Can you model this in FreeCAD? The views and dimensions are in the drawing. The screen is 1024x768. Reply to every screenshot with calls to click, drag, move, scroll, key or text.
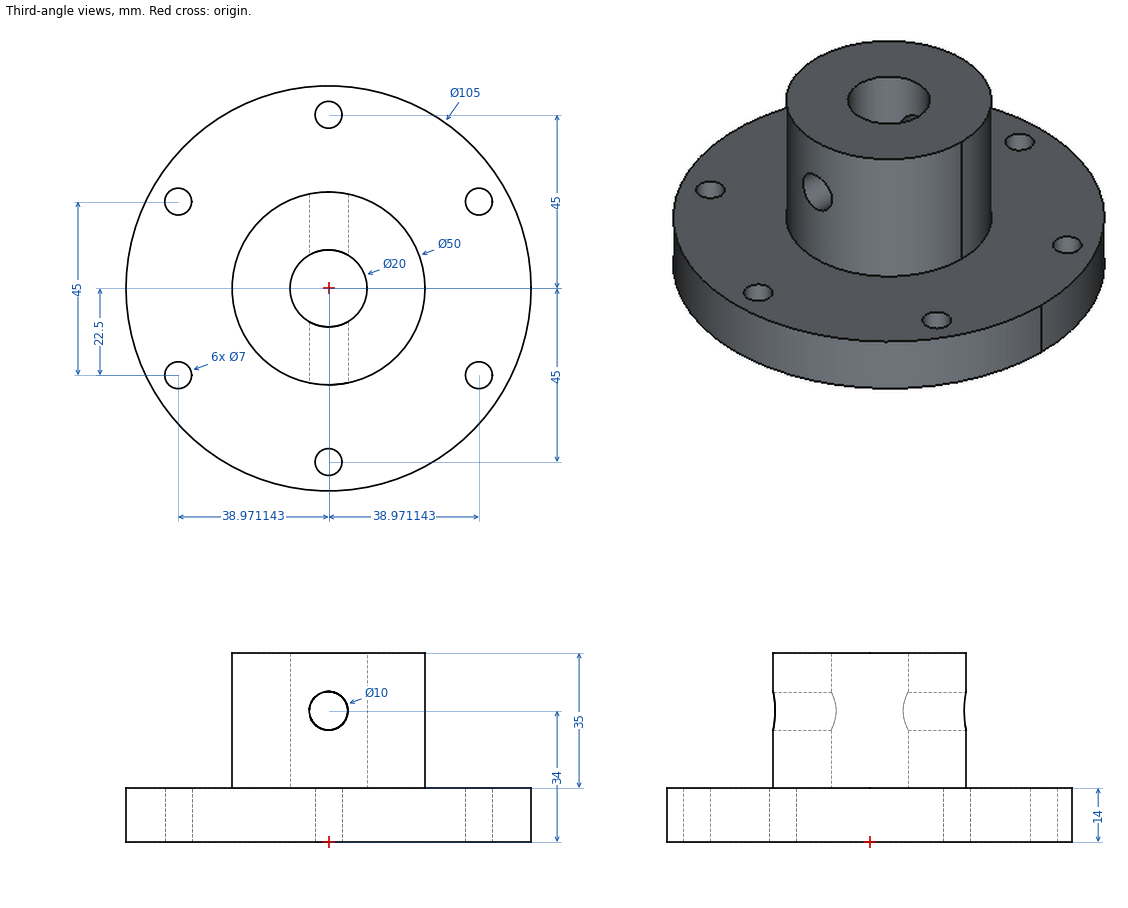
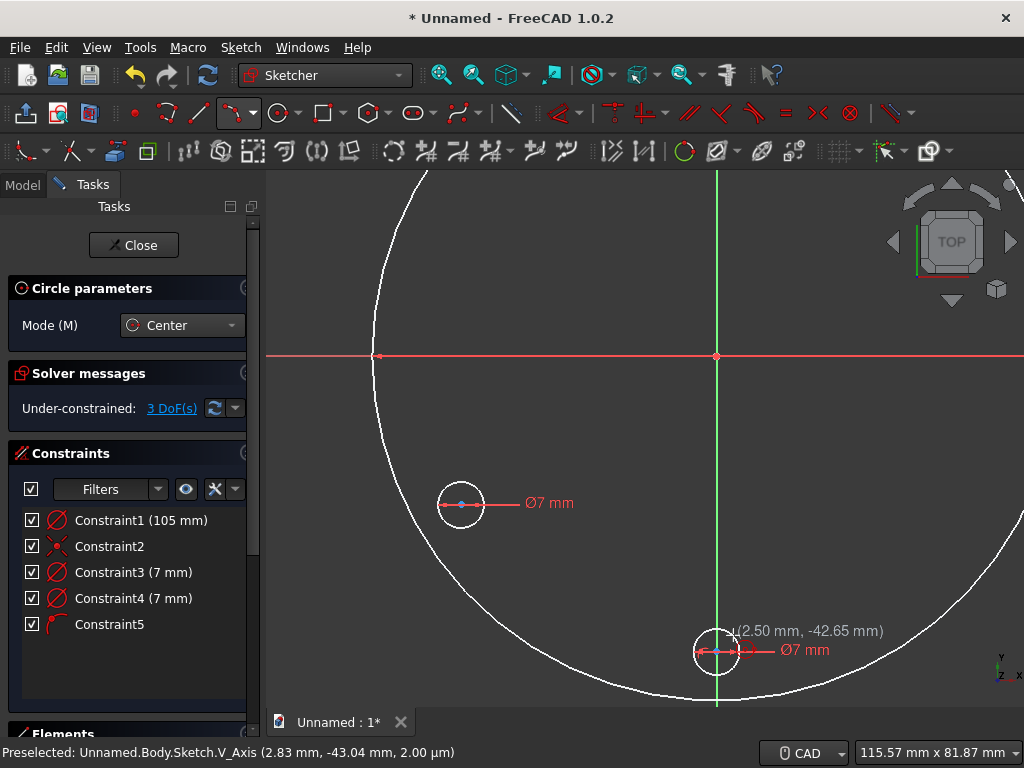
scroll(462, 506, down, 4)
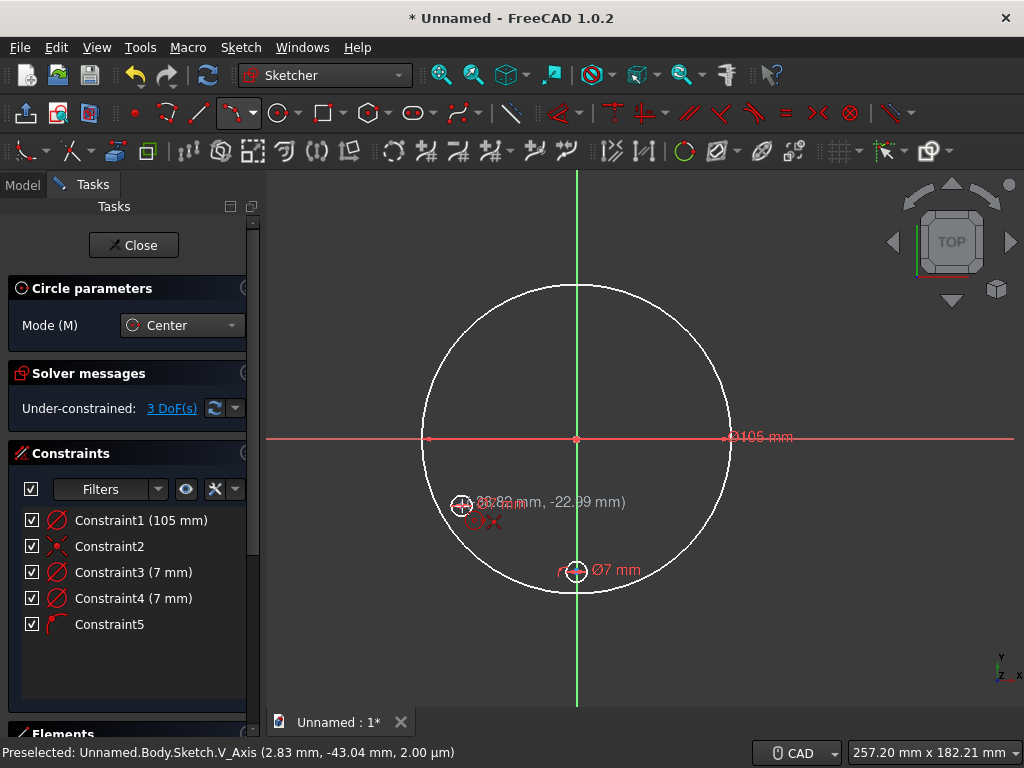
scroll(691, 505, up, 4)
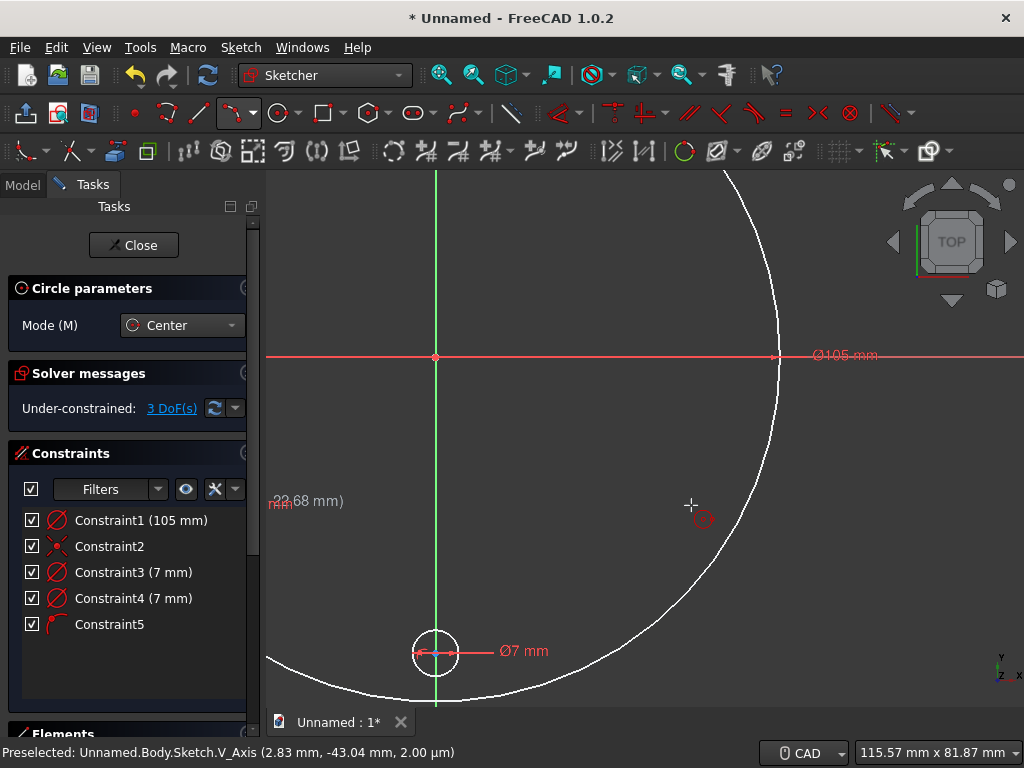
click(691, 505)
move(707, 489)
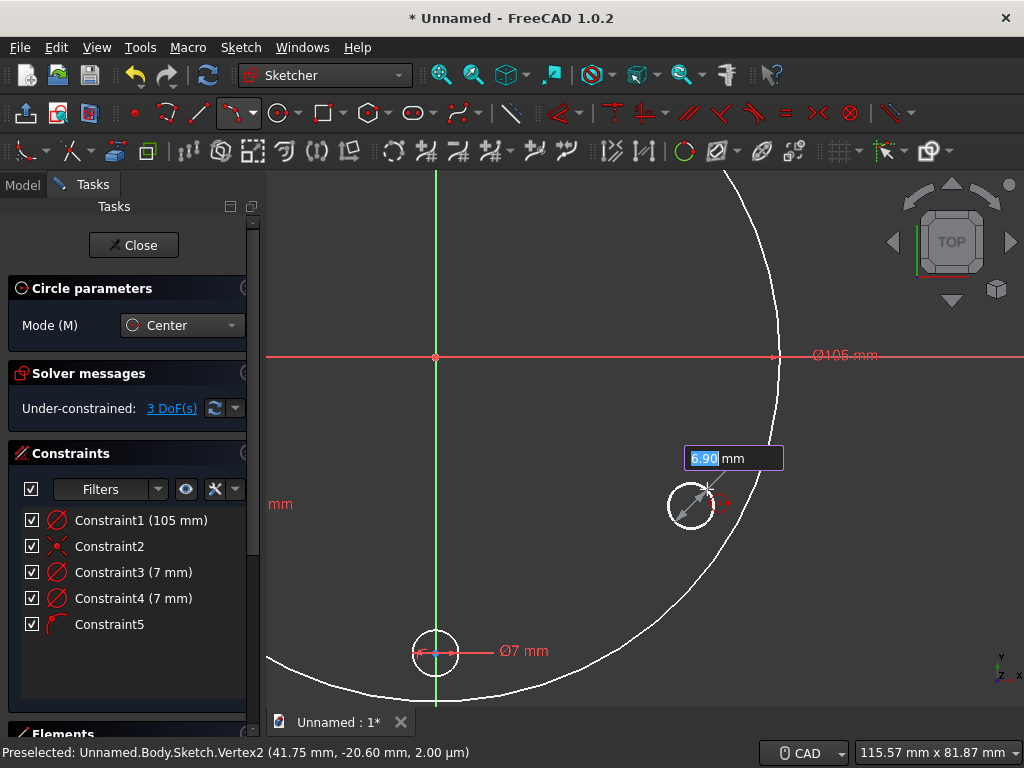
text(7)
key(Return)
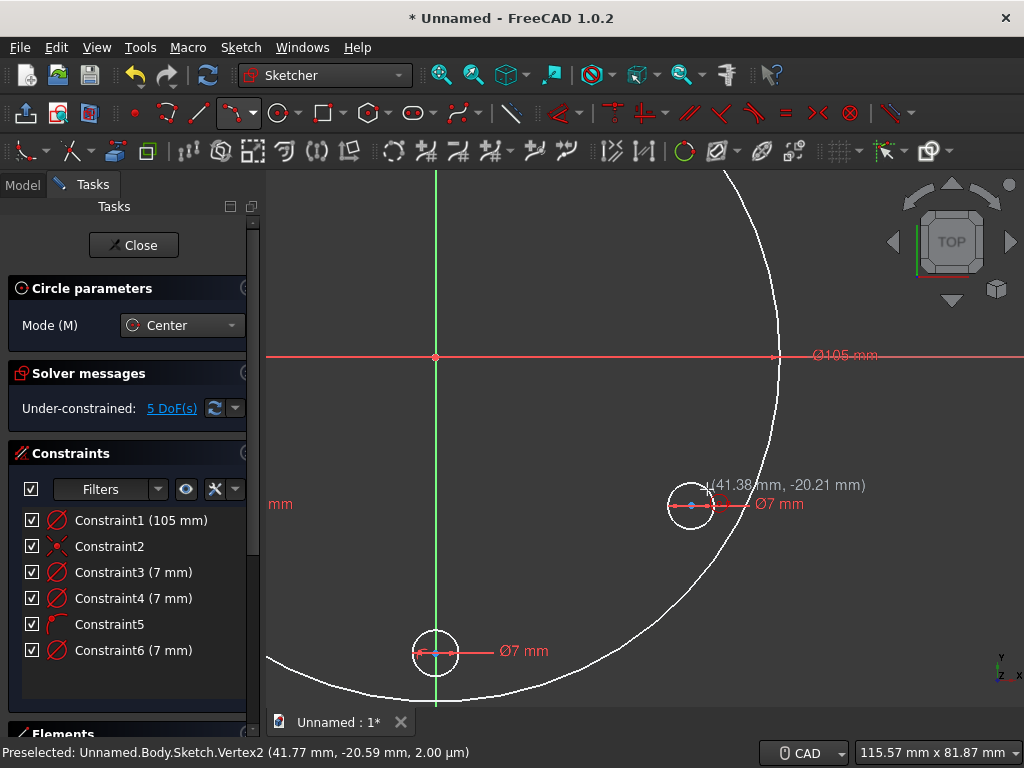
scroll(691, 505, down, 4)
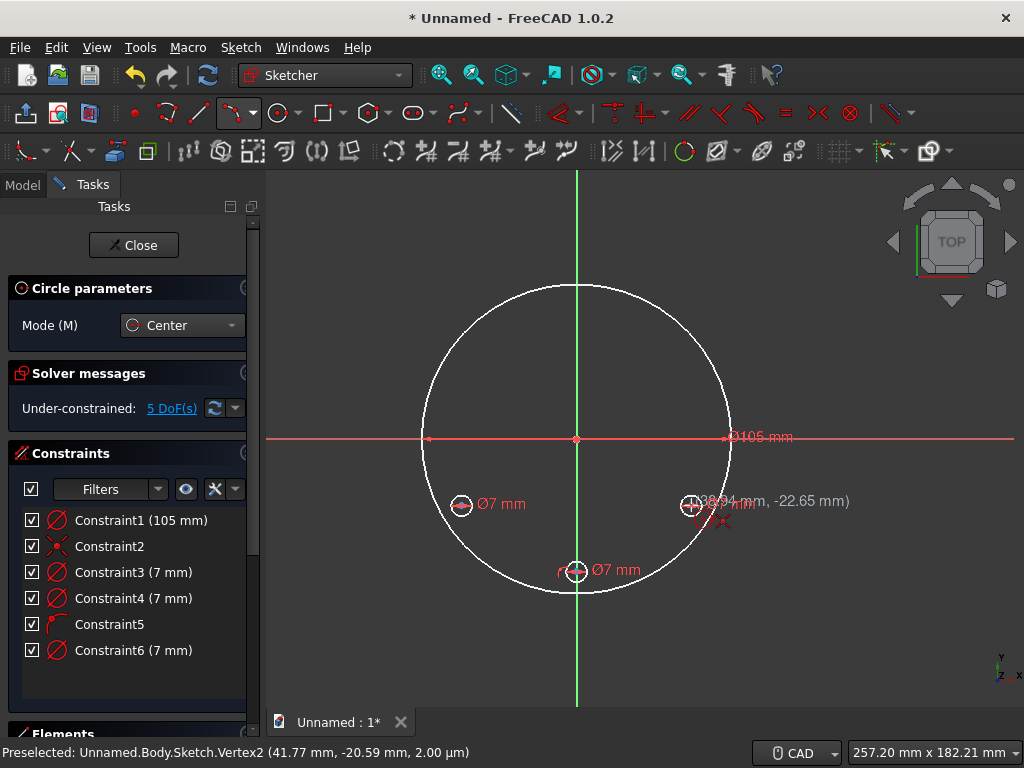
scroll(462, 373, up, 4)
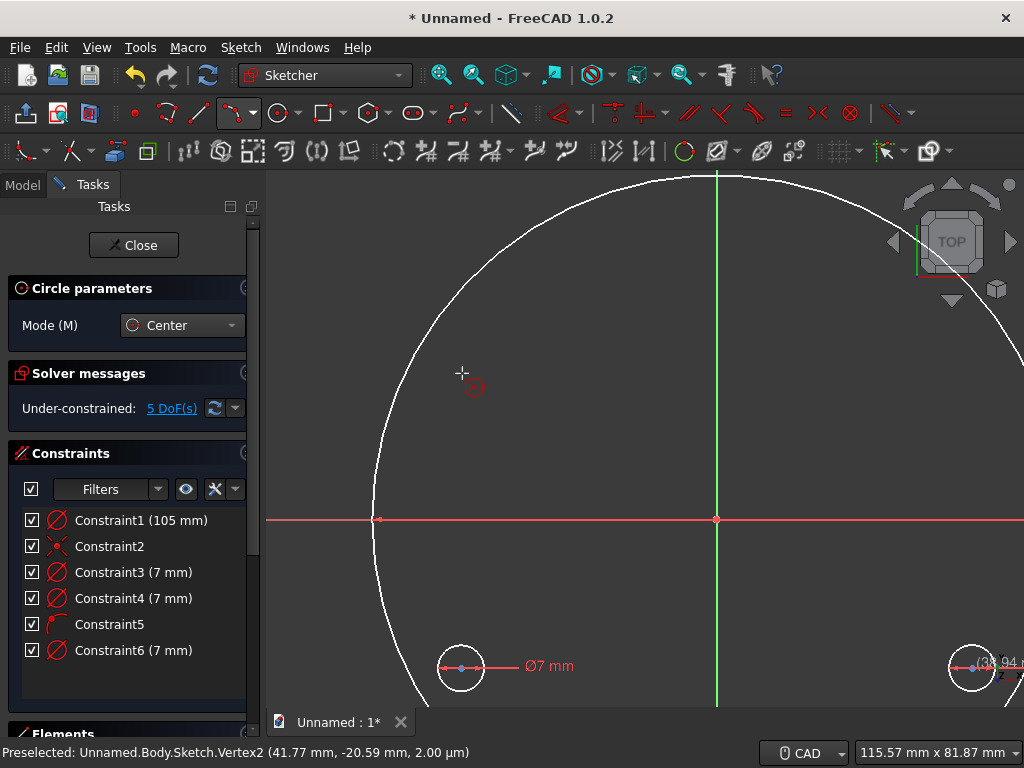
click(461, 372)
move(477, 356)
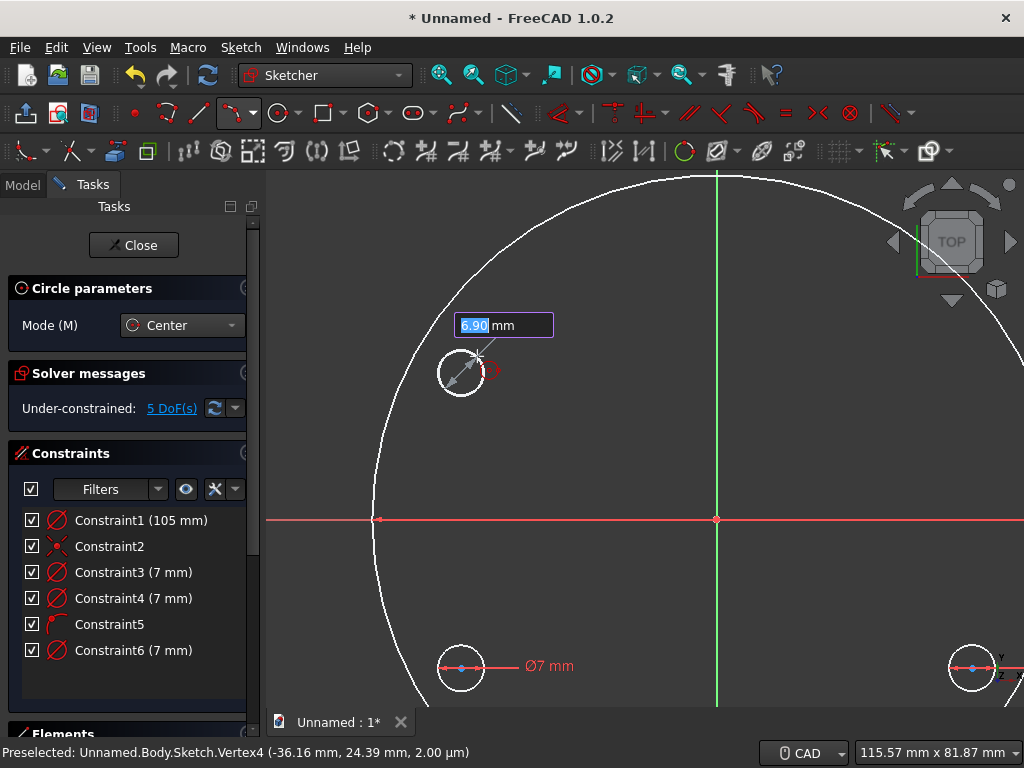
text(7)
key(Return)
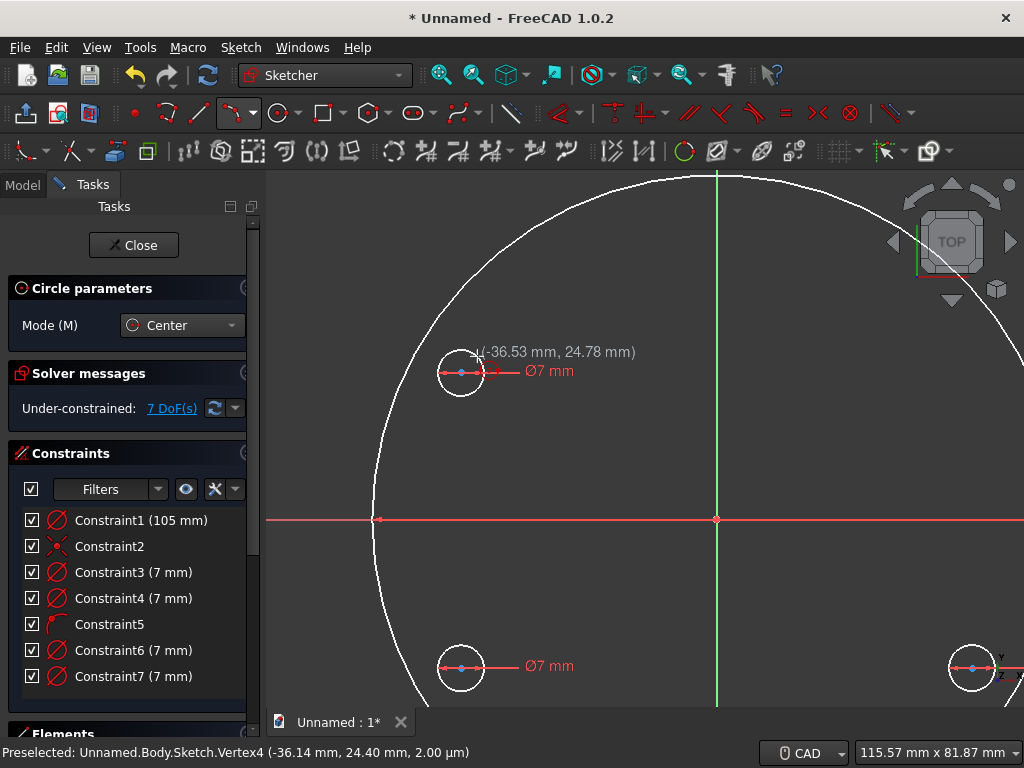
scroll(462, 372, down, 4)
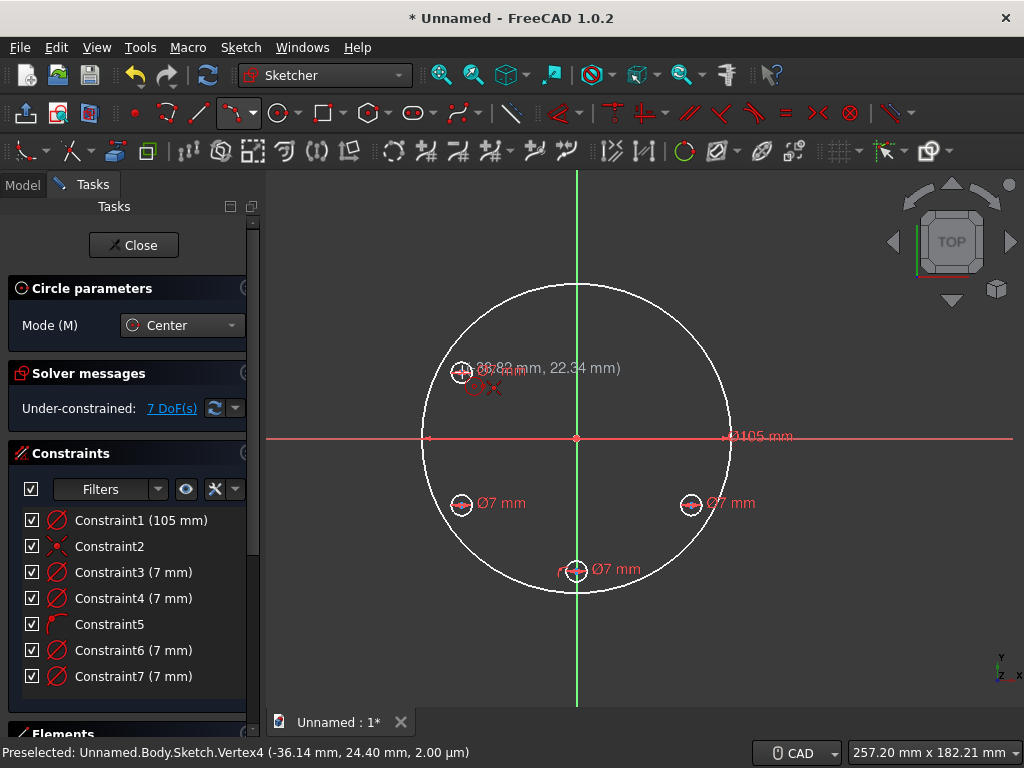
scroll(691, 372, up, 4)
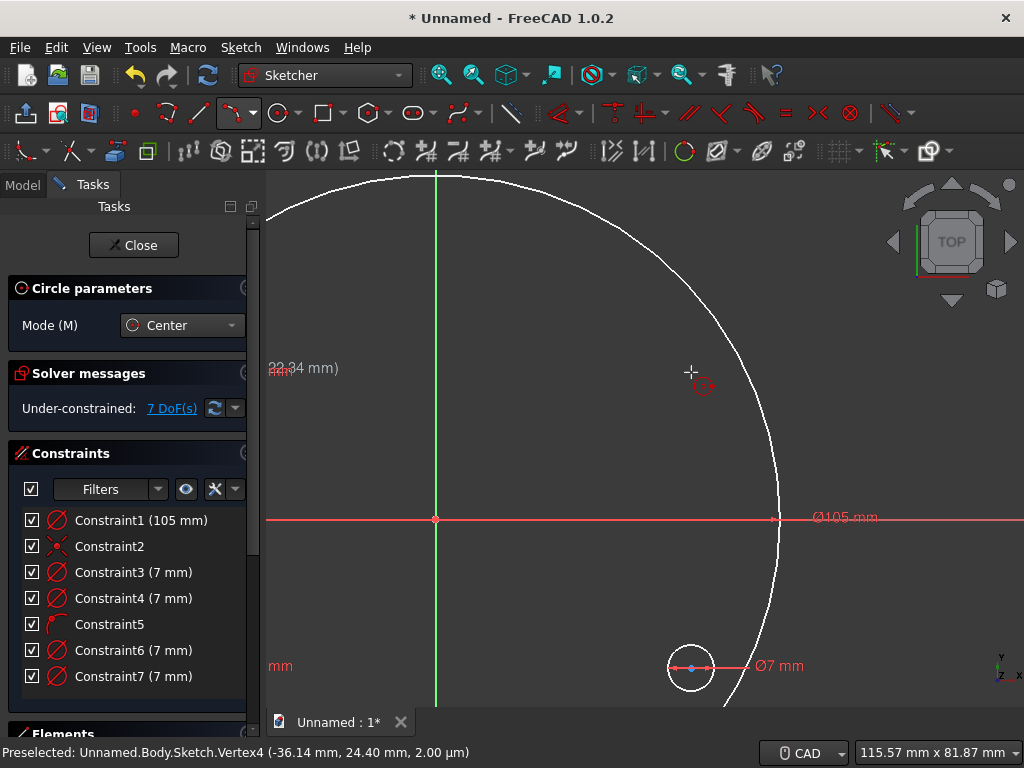
click(691, 372)
move(707, 356)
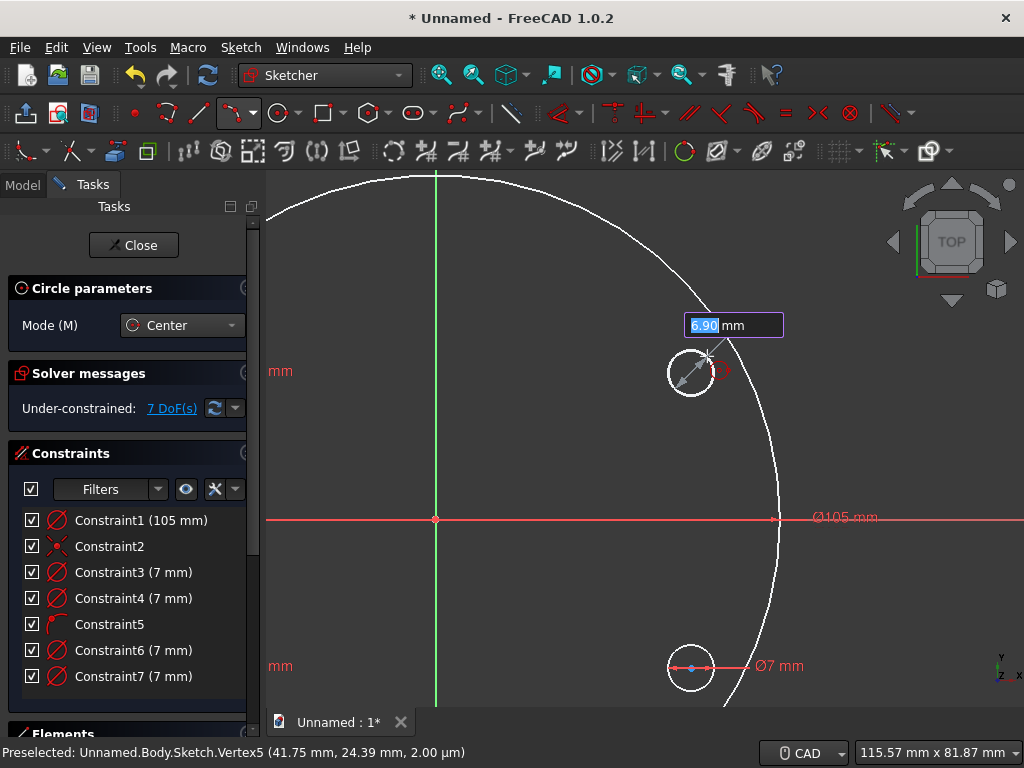
text(7)
key(Return)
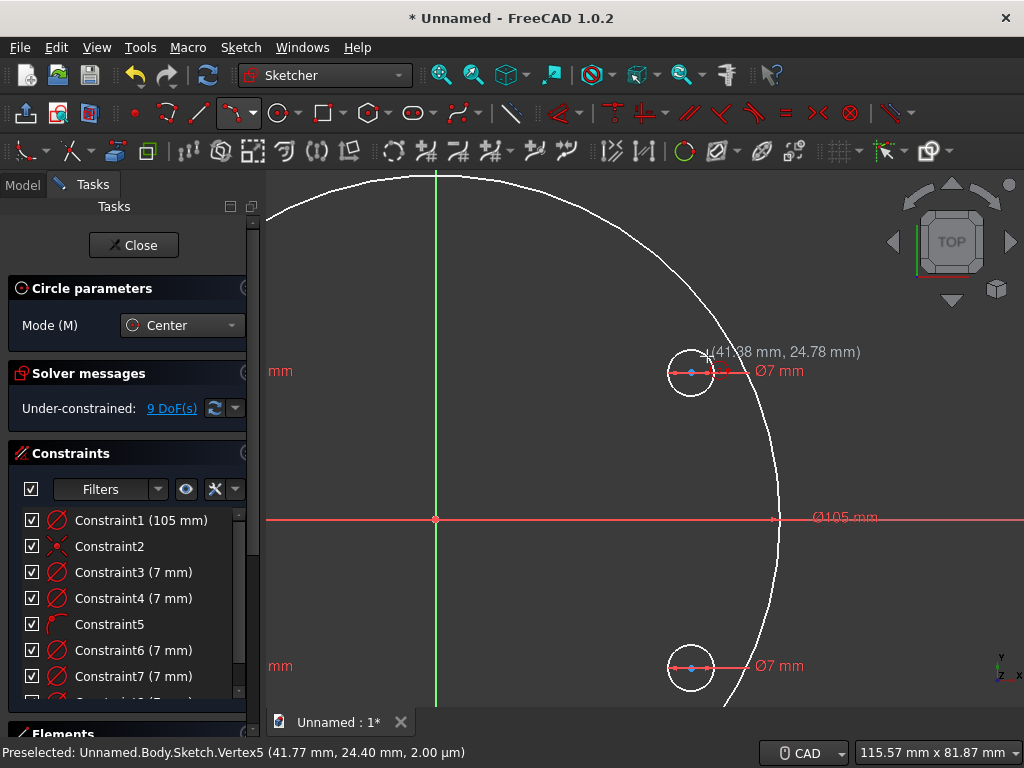
click(436, 224)
move(452, 208)